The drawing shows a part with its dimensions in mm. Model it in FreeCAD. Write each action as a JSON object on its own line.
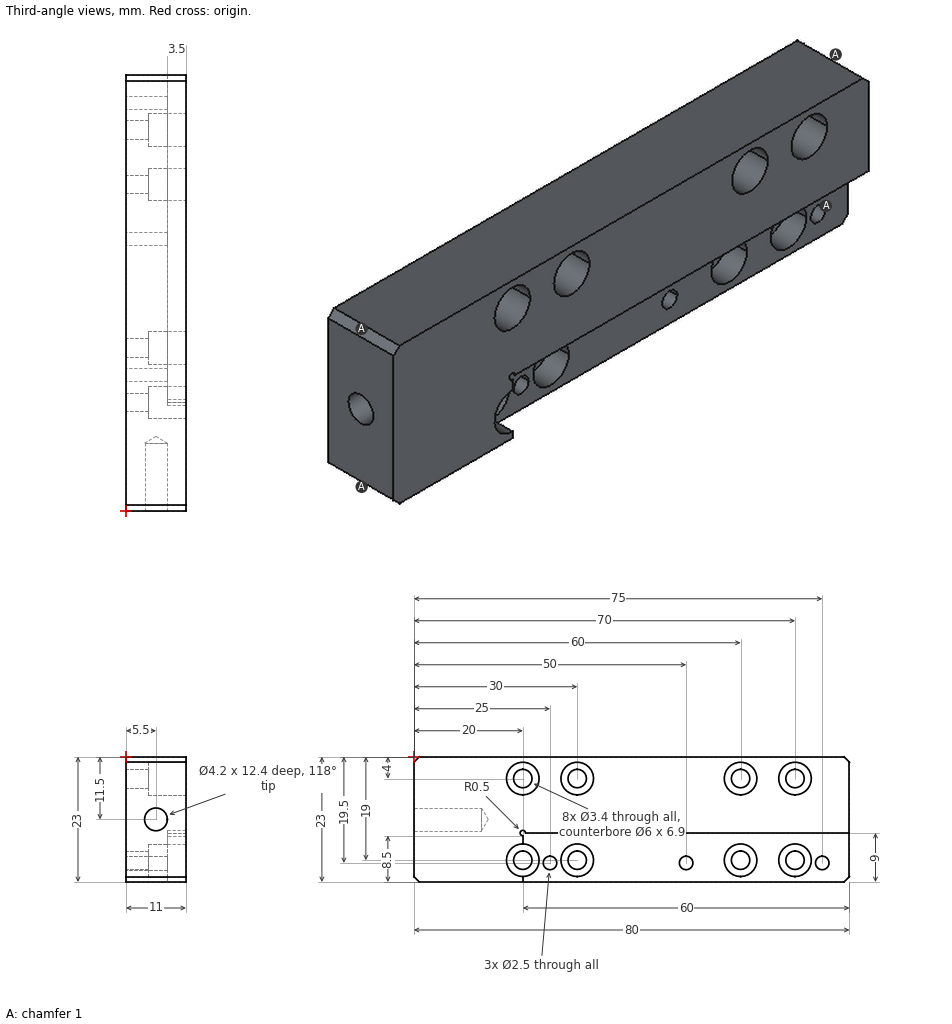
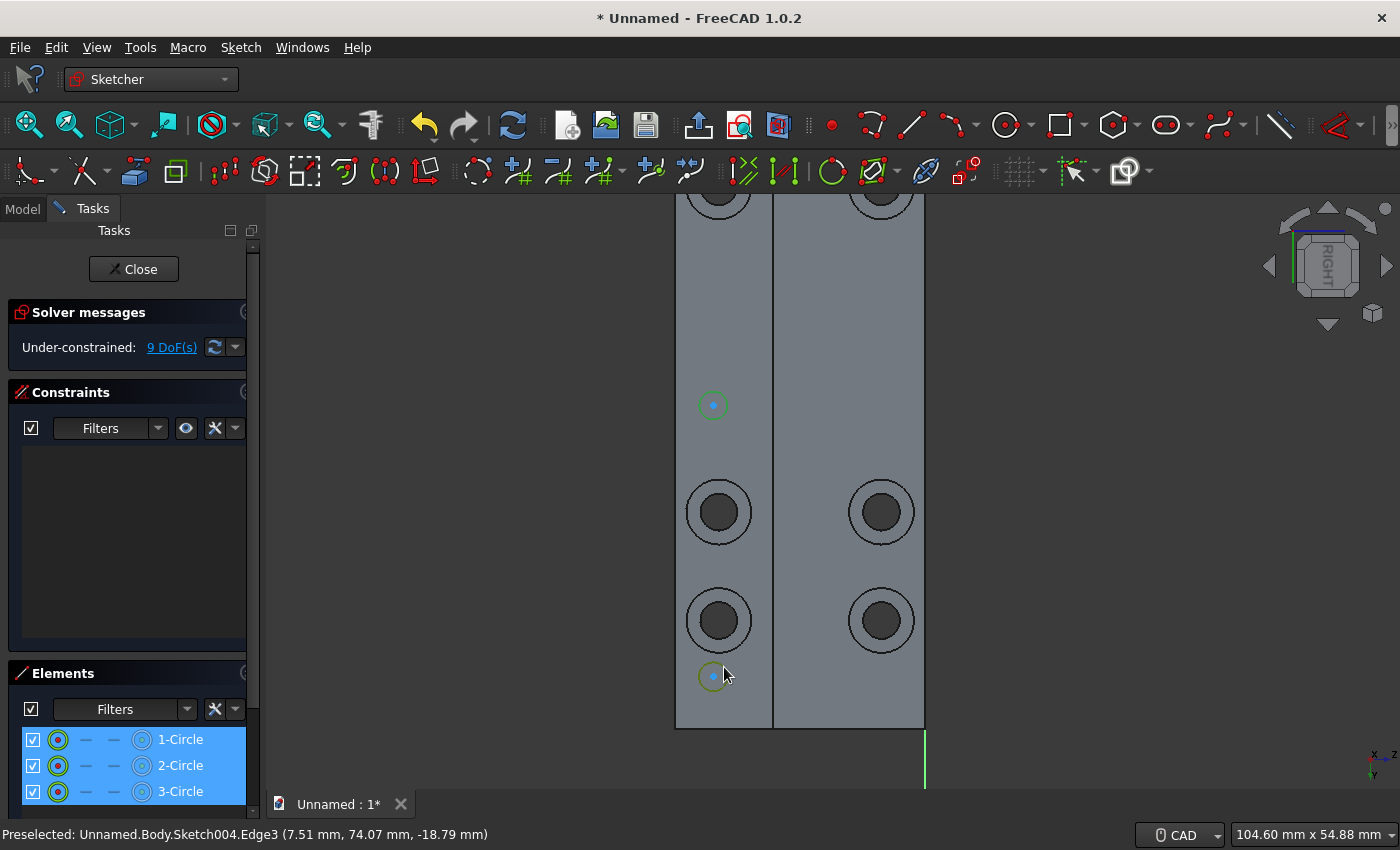
{"action": "key", "text": "e"}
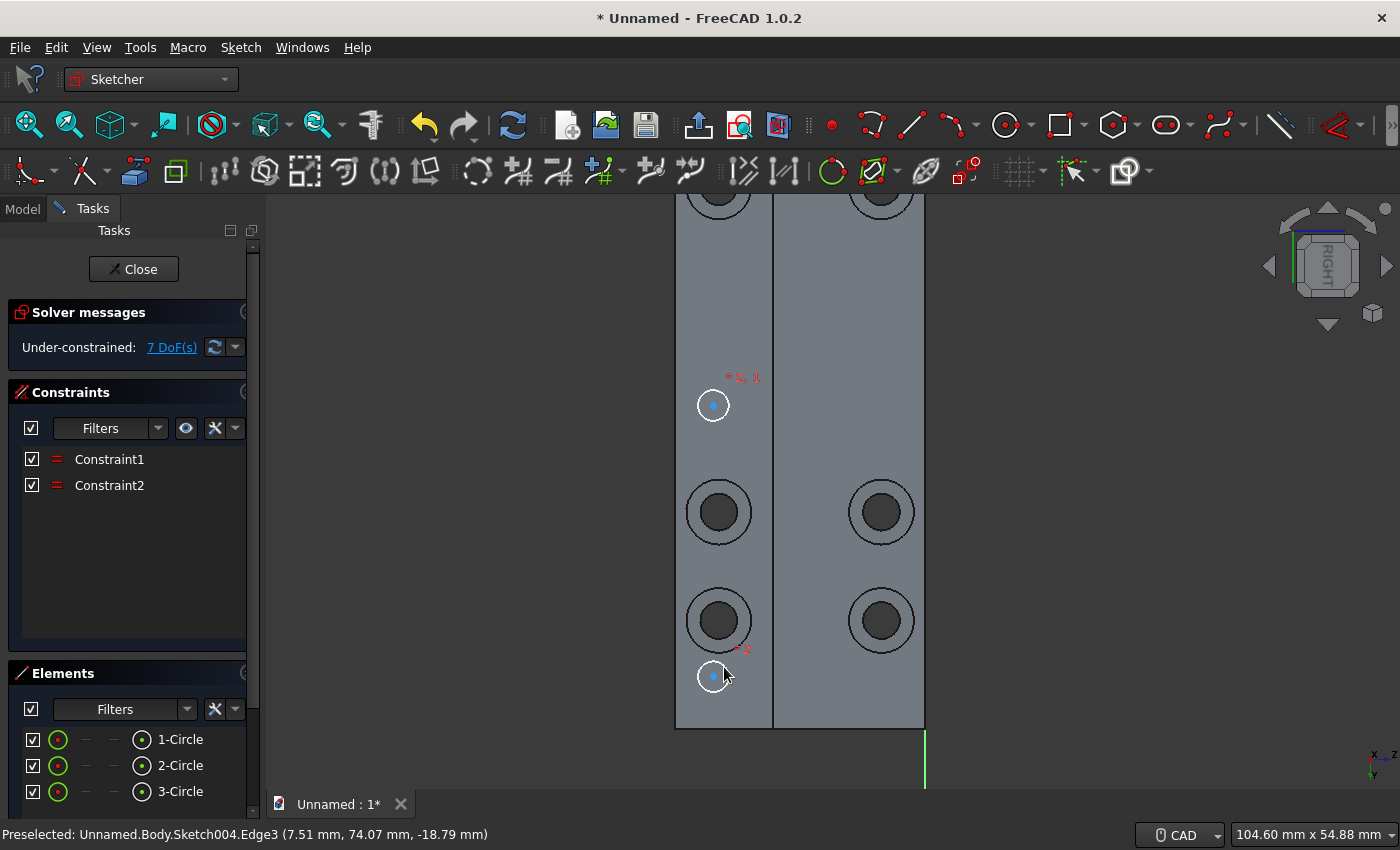
{"action": "scroll", "coordinate": [725, 668], "scroll_direction": "down", "scroll_amount": 4}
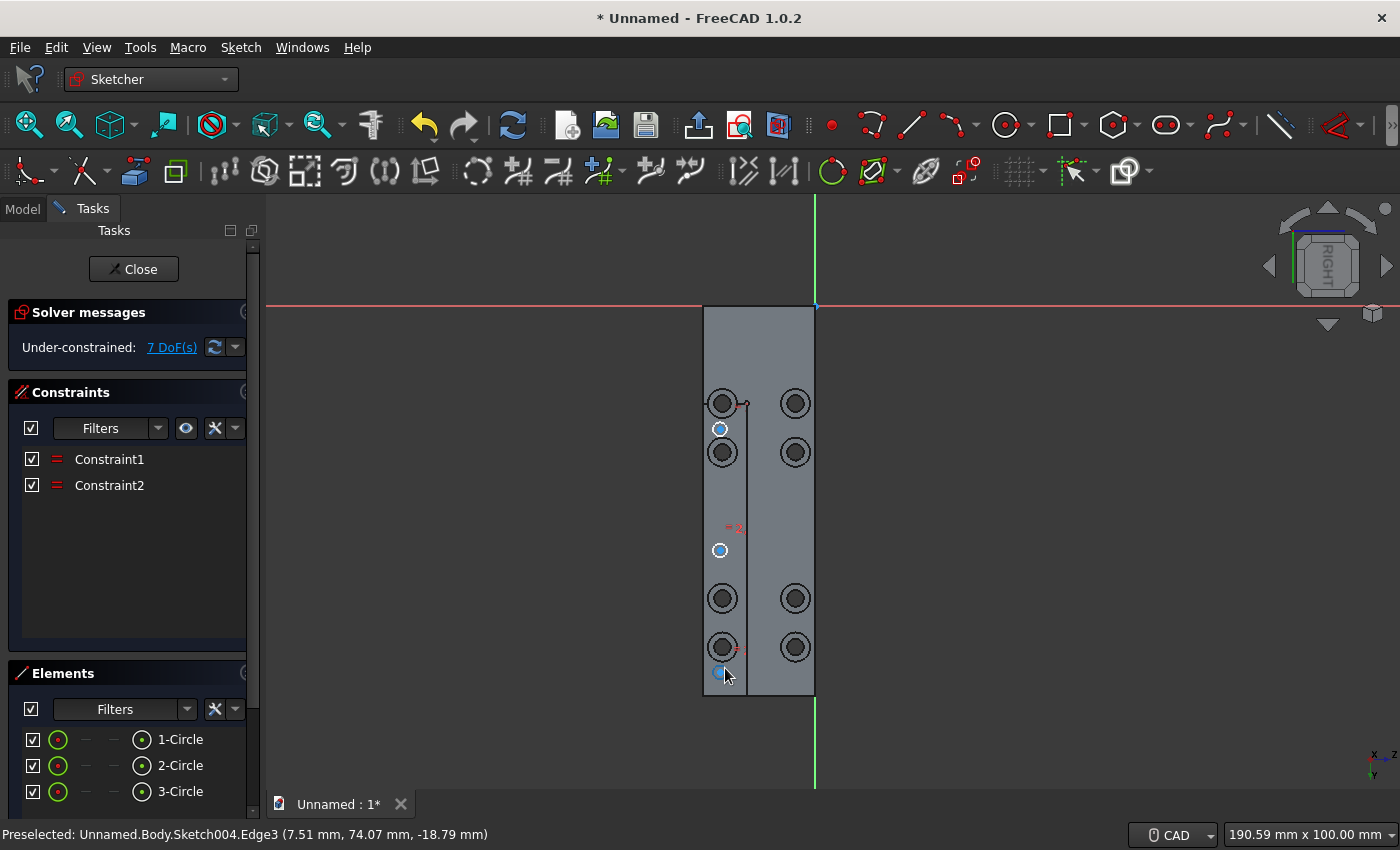
{"action": "left_click", "coordinate": [720, 429]}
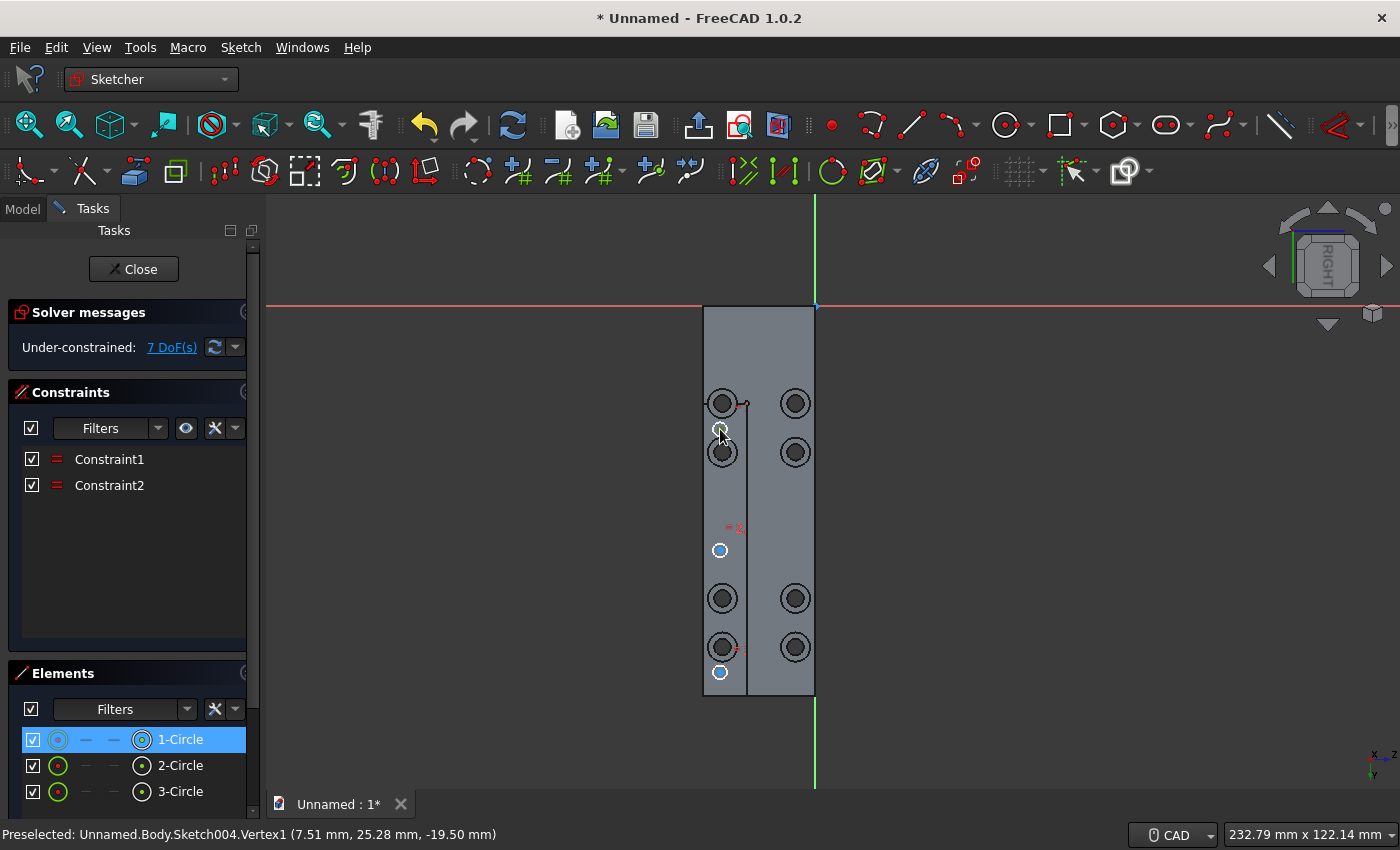
{"action": "left_click", "coordinate": [720, 550]}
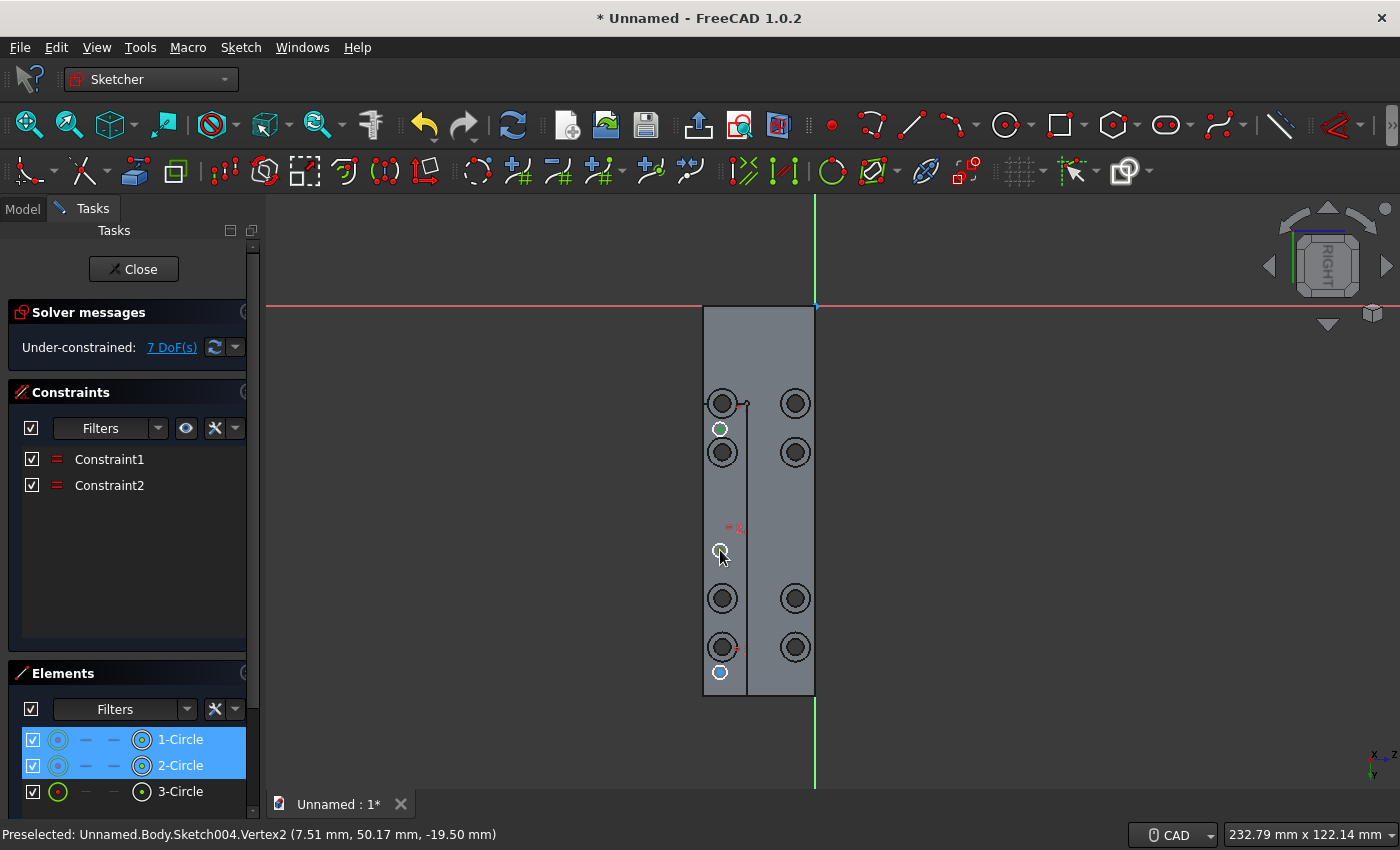
{"action": "key", "text": "v"}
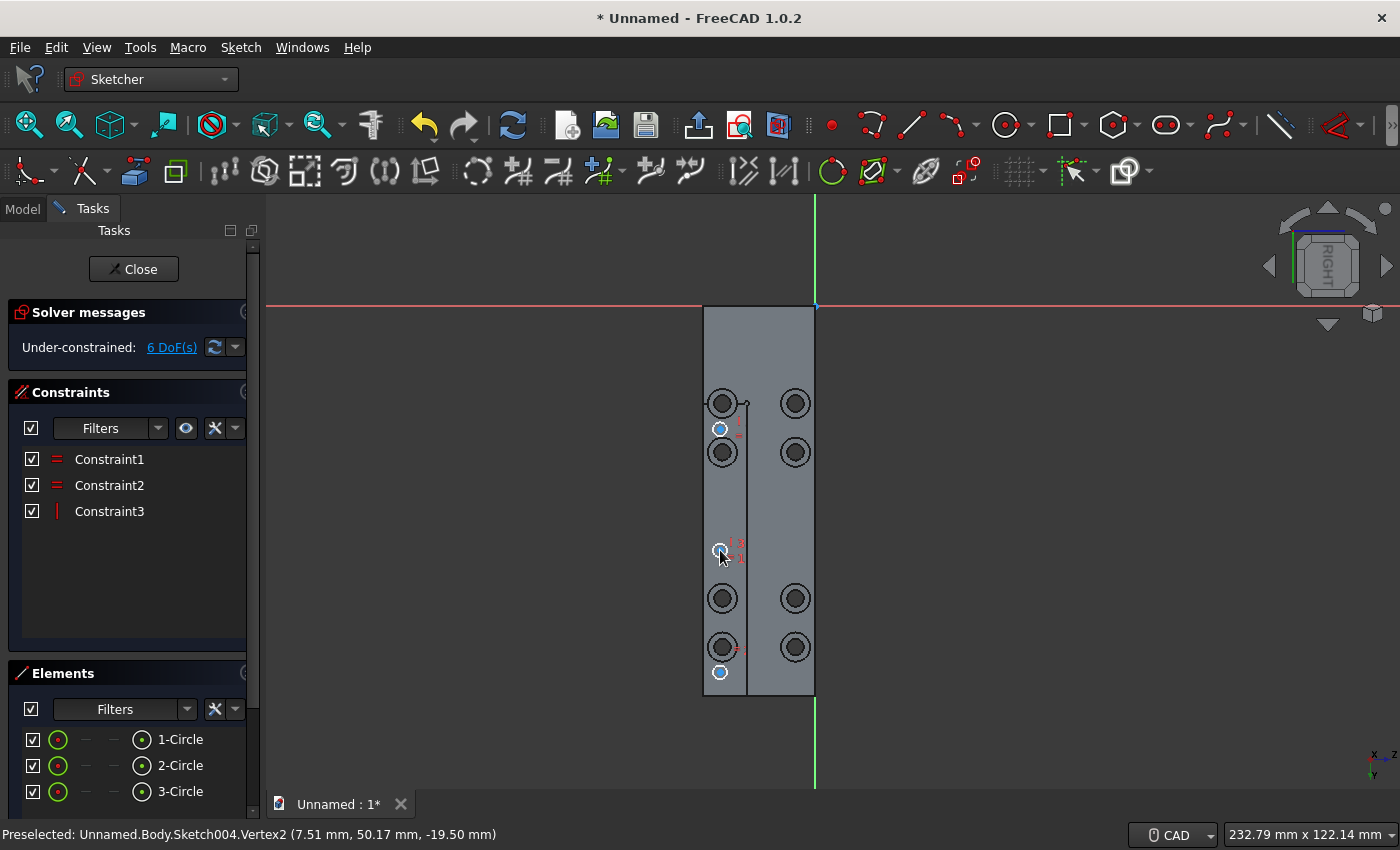
{"action": "left_click", "coordinate": [720, 550]}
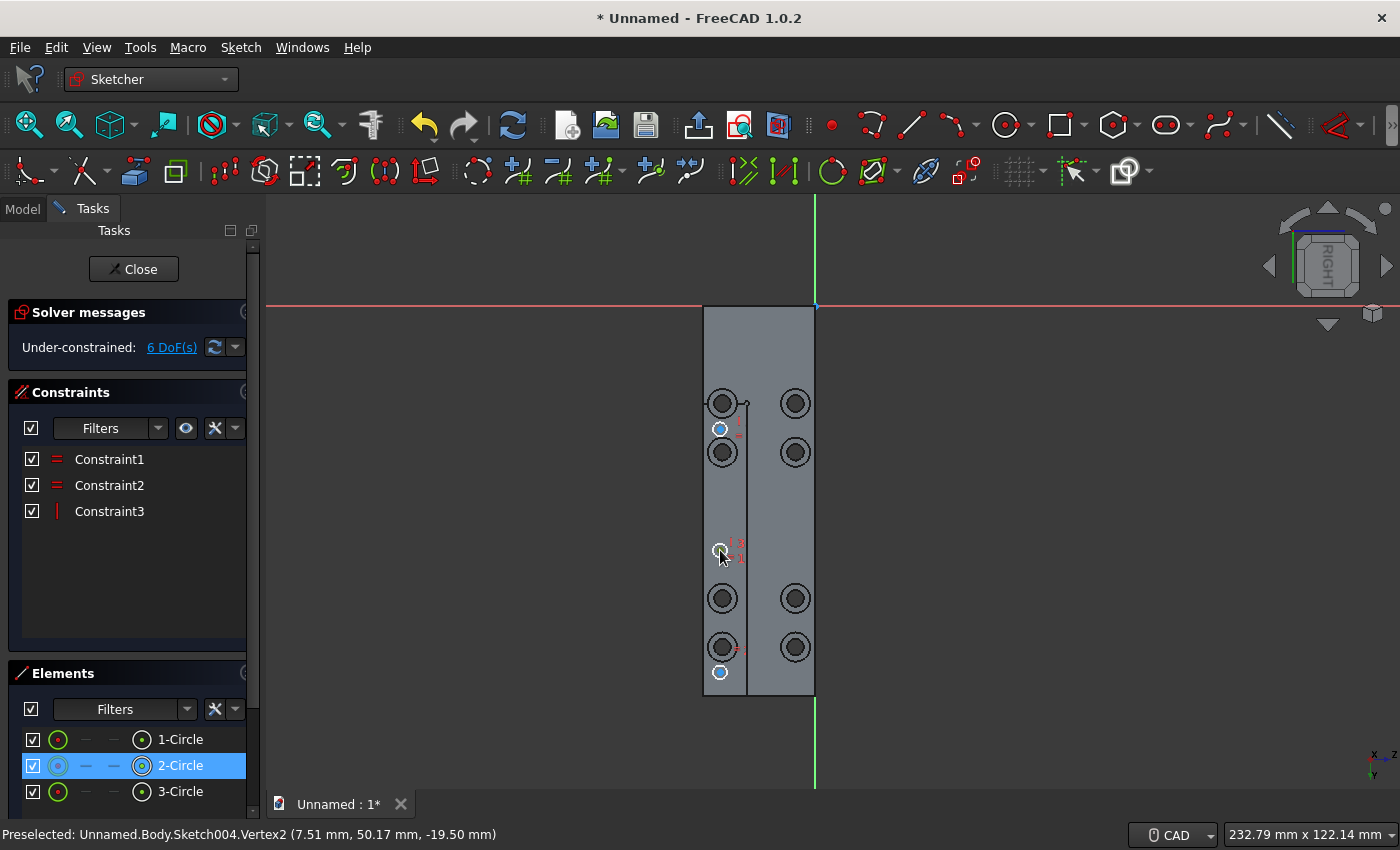
{"action": "left_click", "coordinate": [720, 672]}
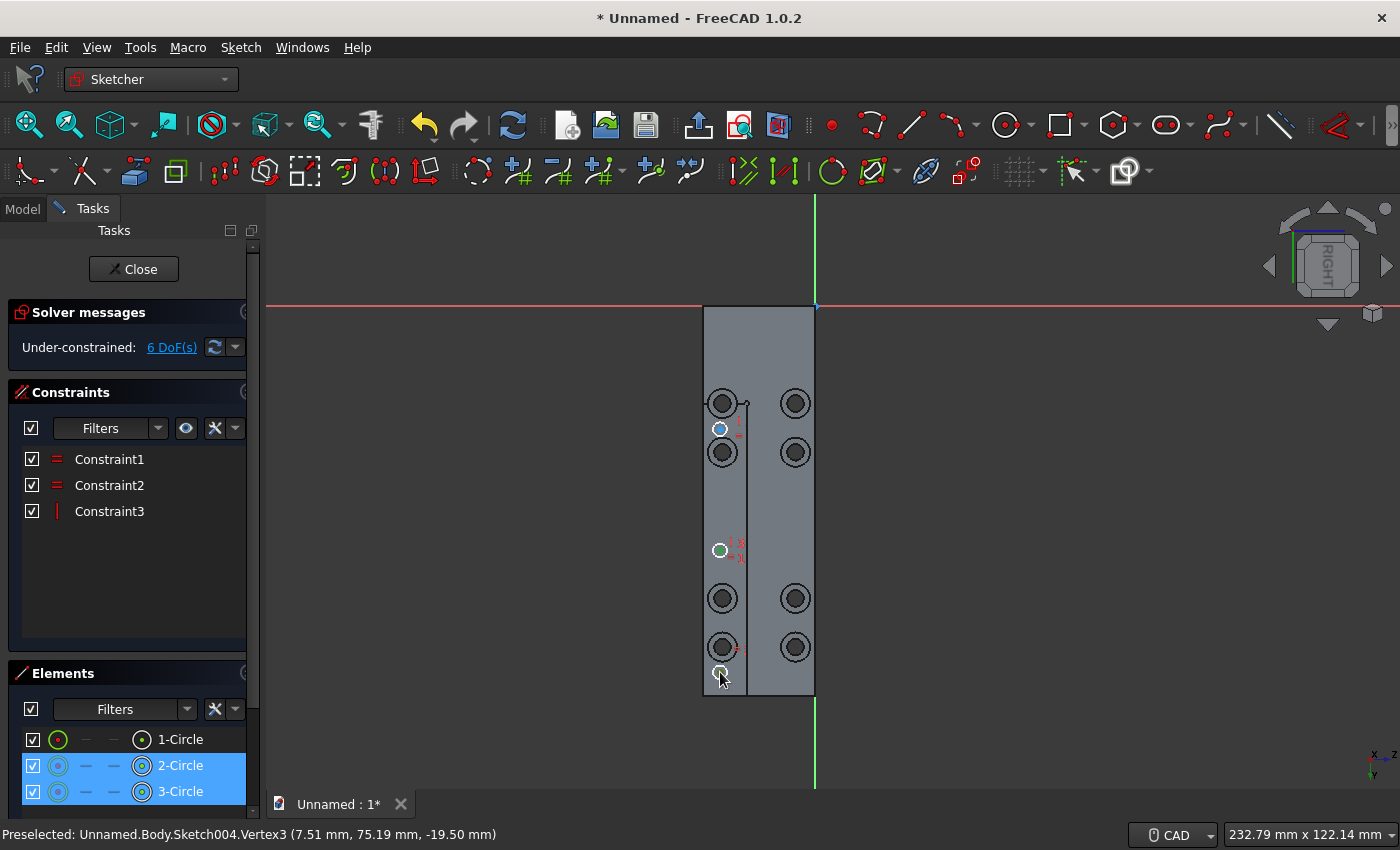
{"action": "key", "text": "v"}